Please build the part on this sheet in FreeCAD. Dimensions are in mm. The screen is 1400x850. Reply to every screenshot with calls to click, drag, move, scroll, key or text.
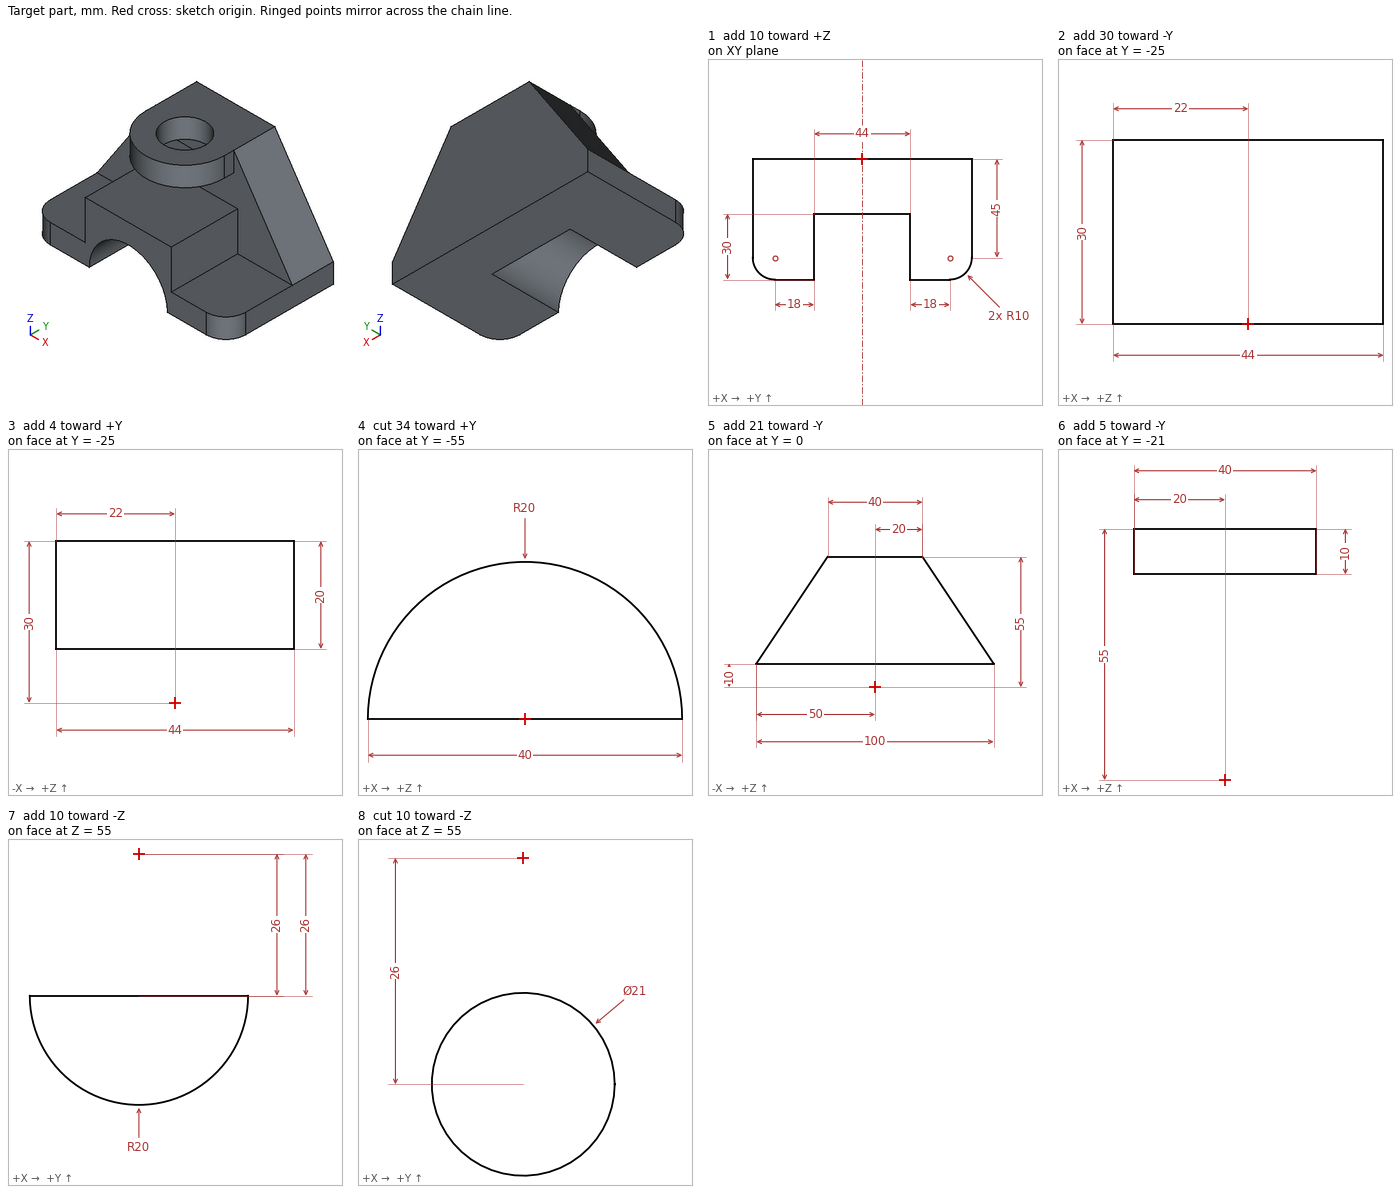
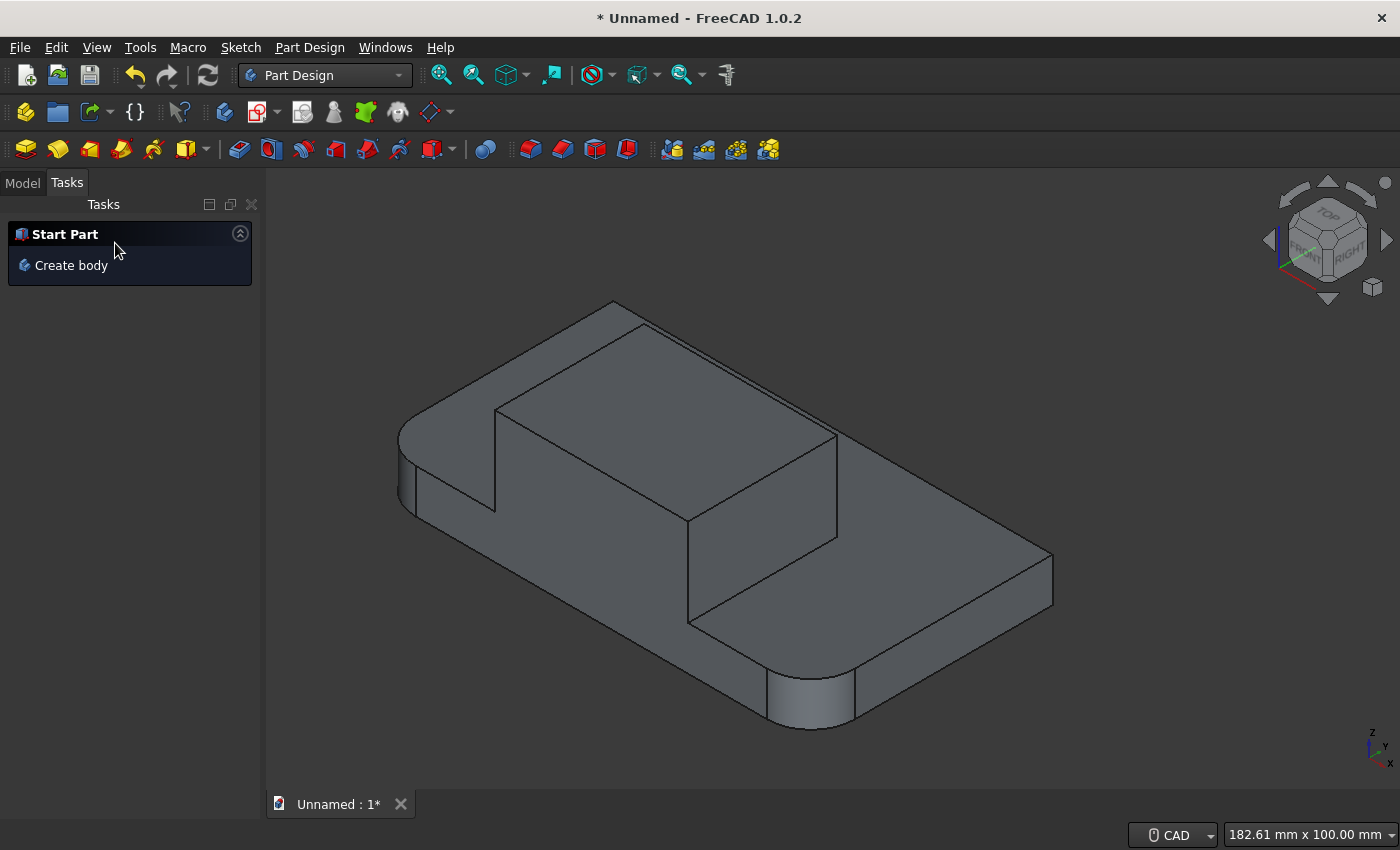
click(591, 541)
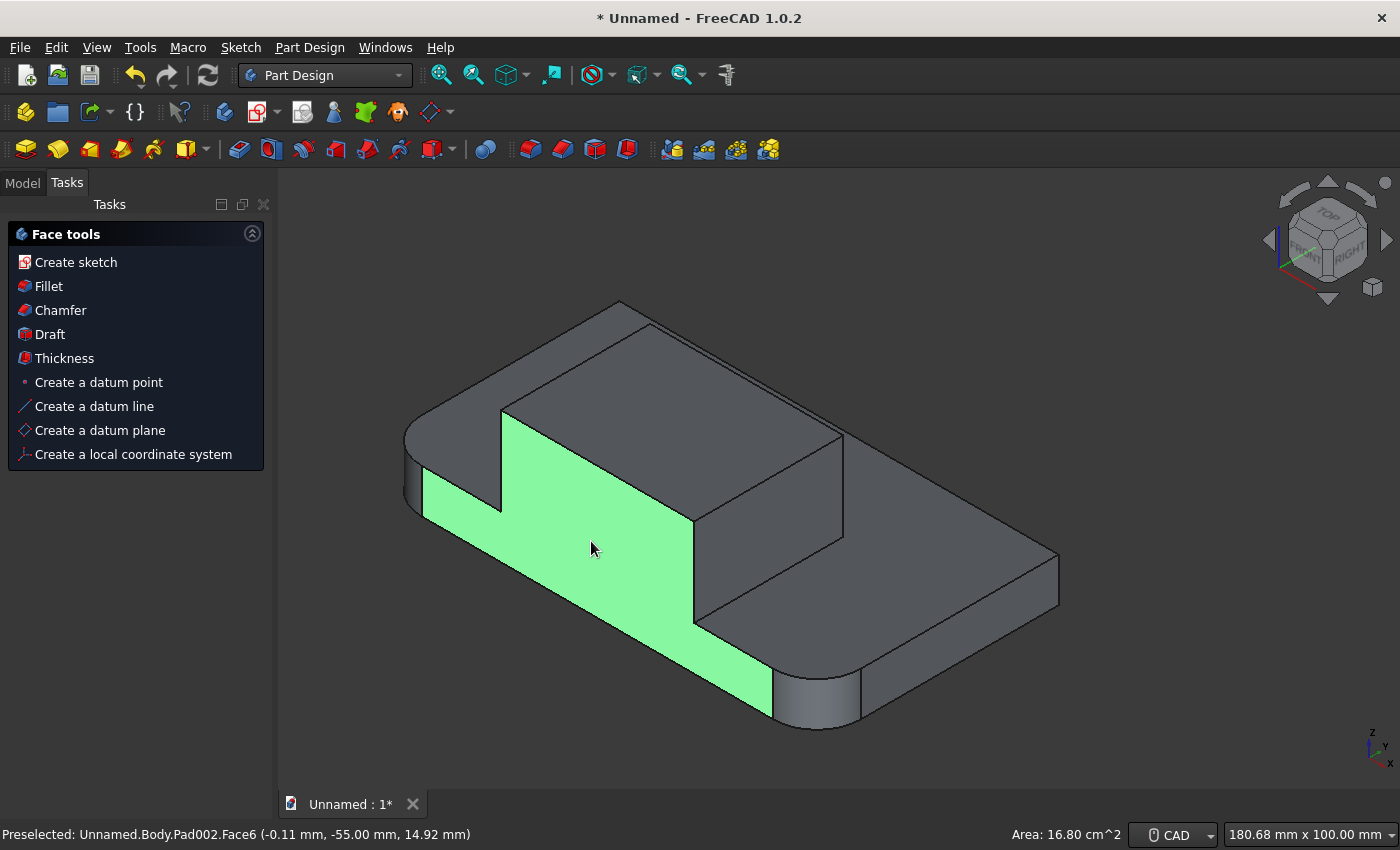
click(258, 112)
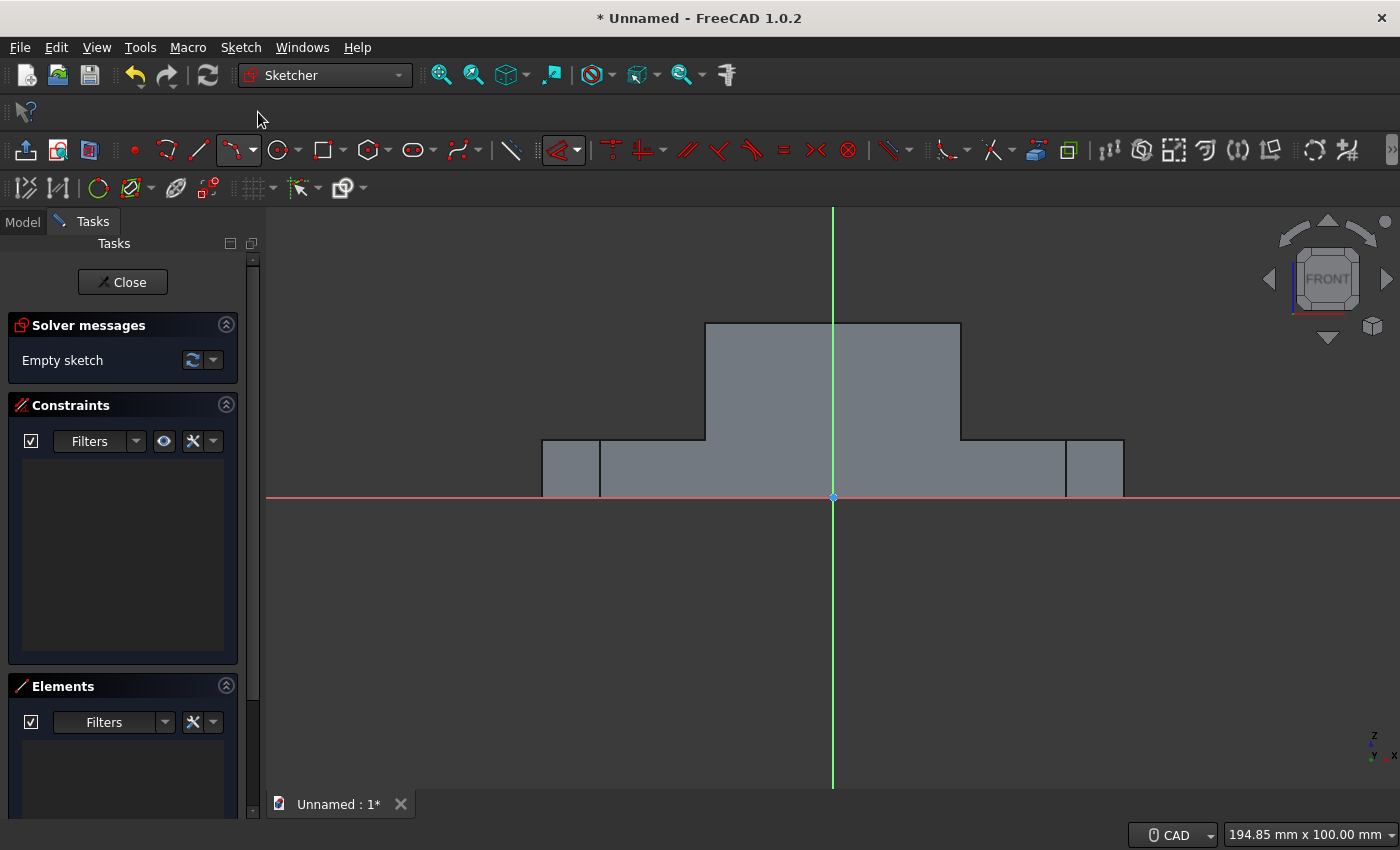
scroll(873, 406, up, 5)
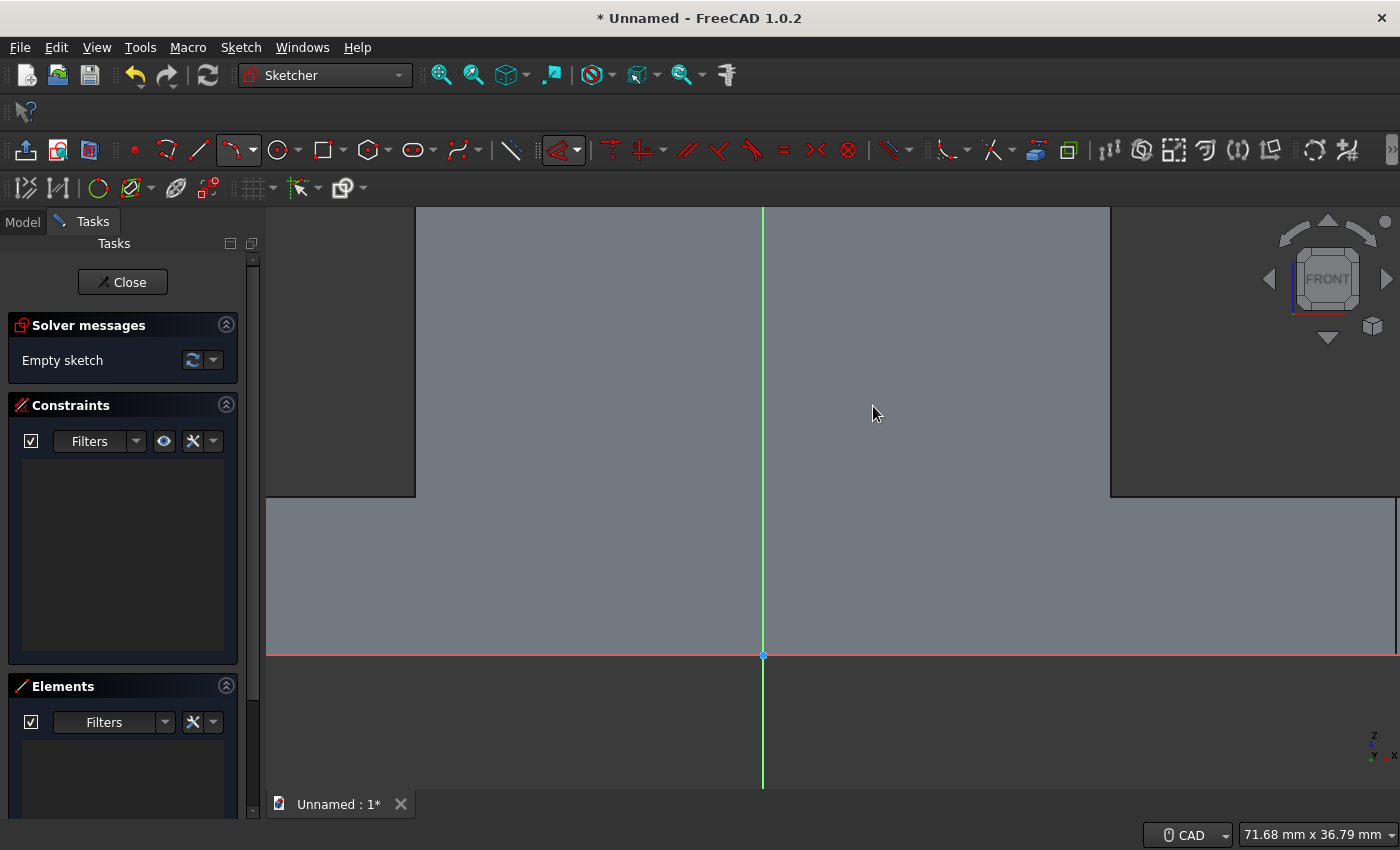
click(200, 150)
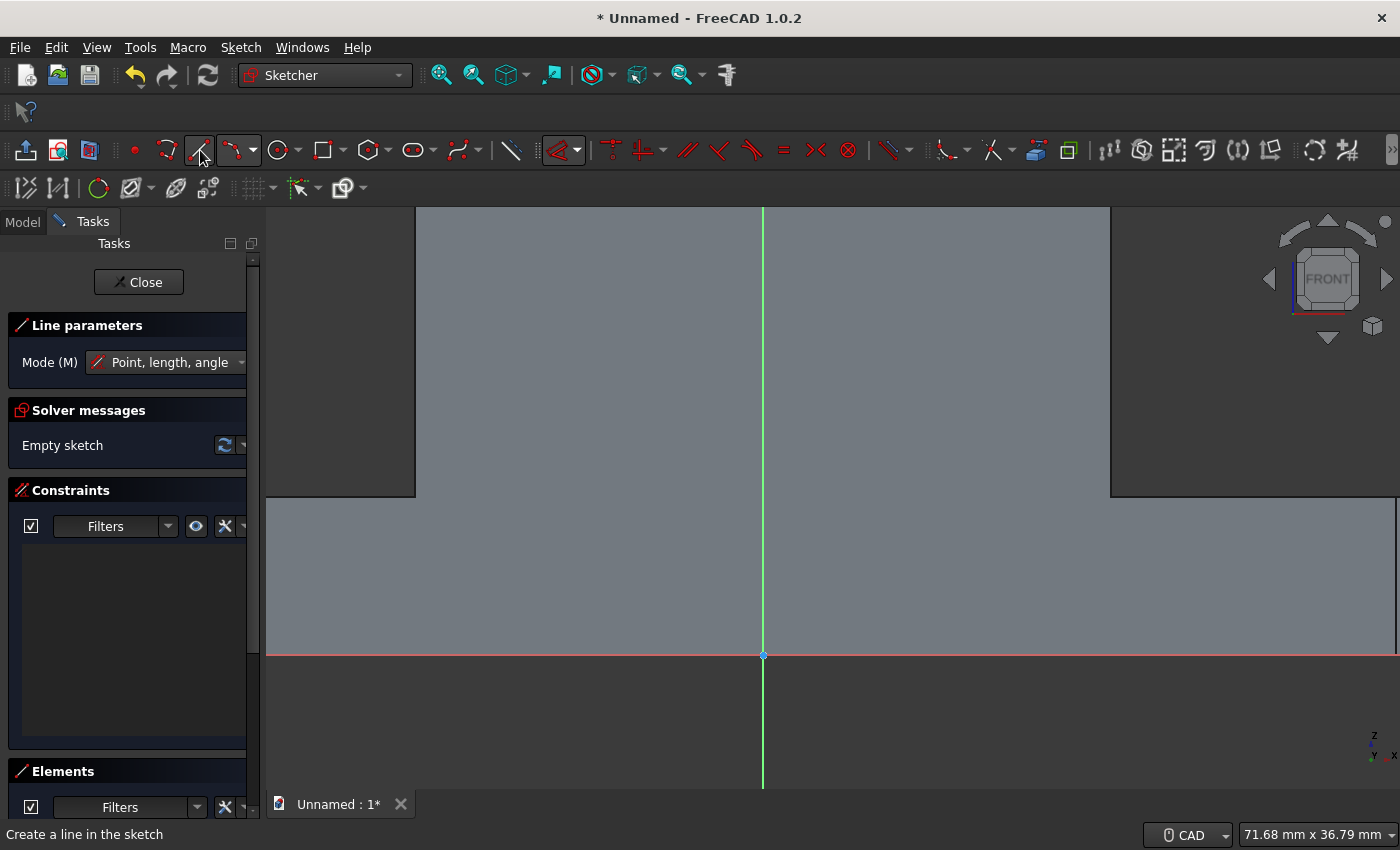
click(447, 655)
click(1080, 646)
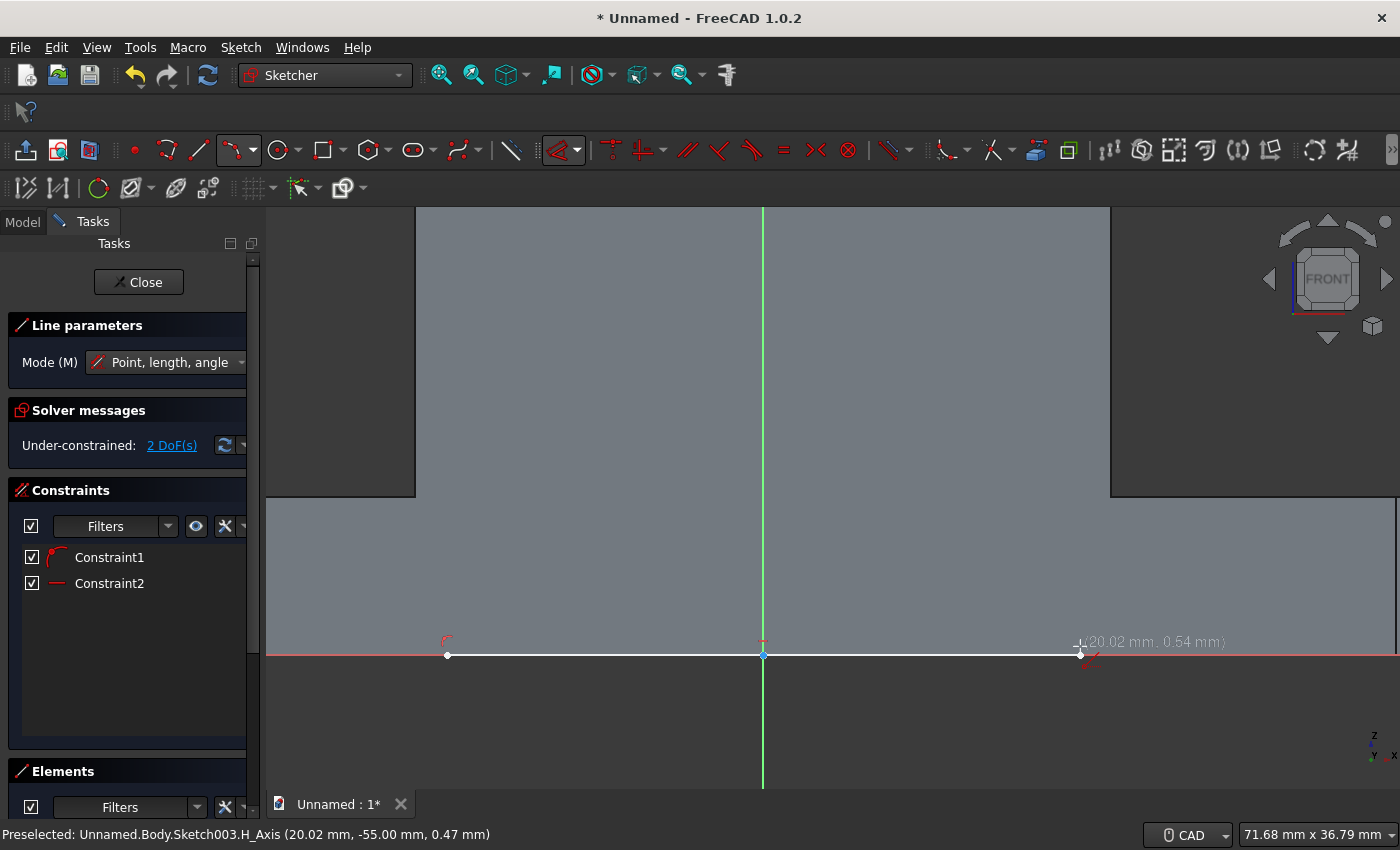
click(232, 150)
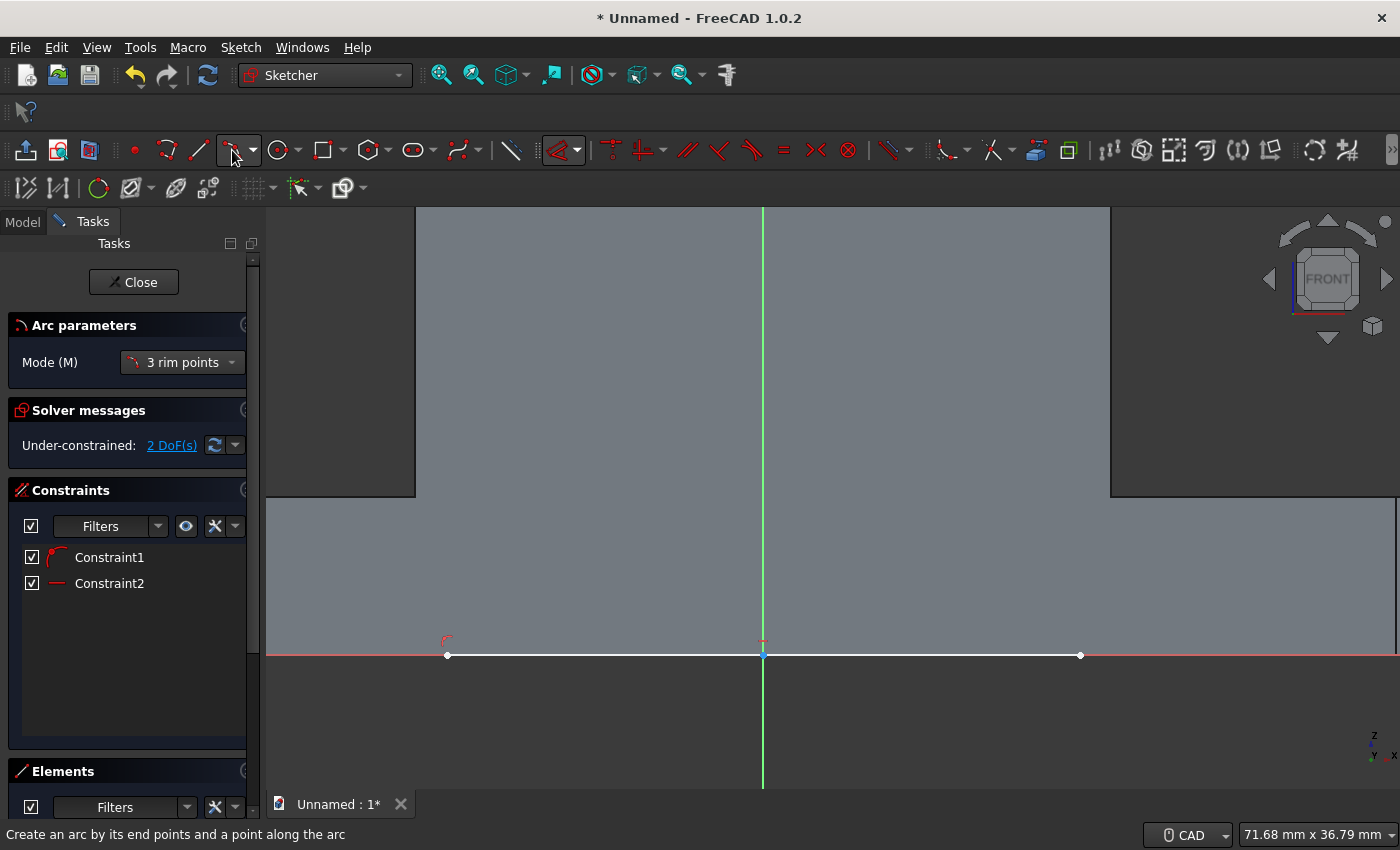
click(1080, 646)
click(447, 655)
click(861, 355)
key(Escape)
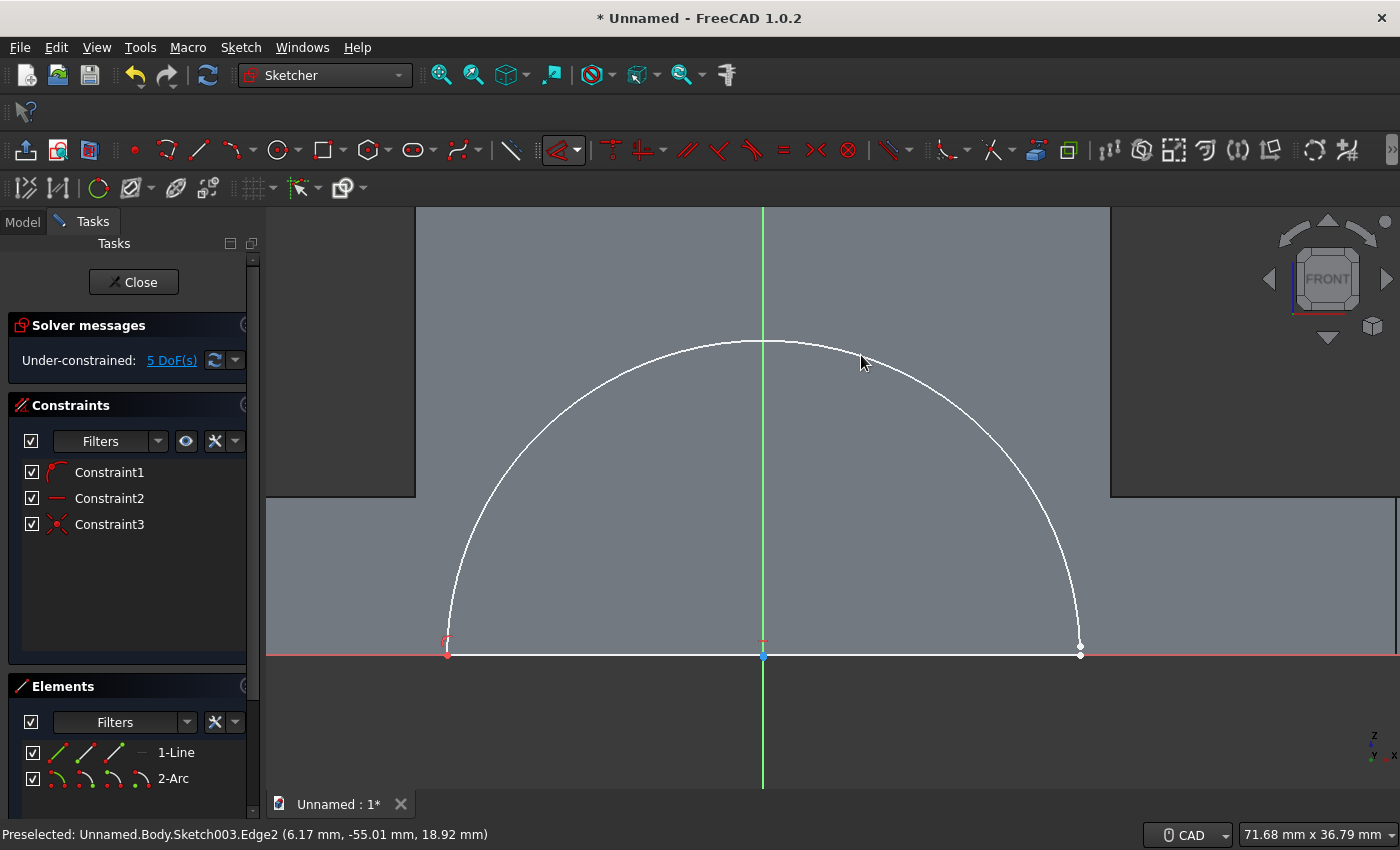
drag(753, 645, 774, 667)